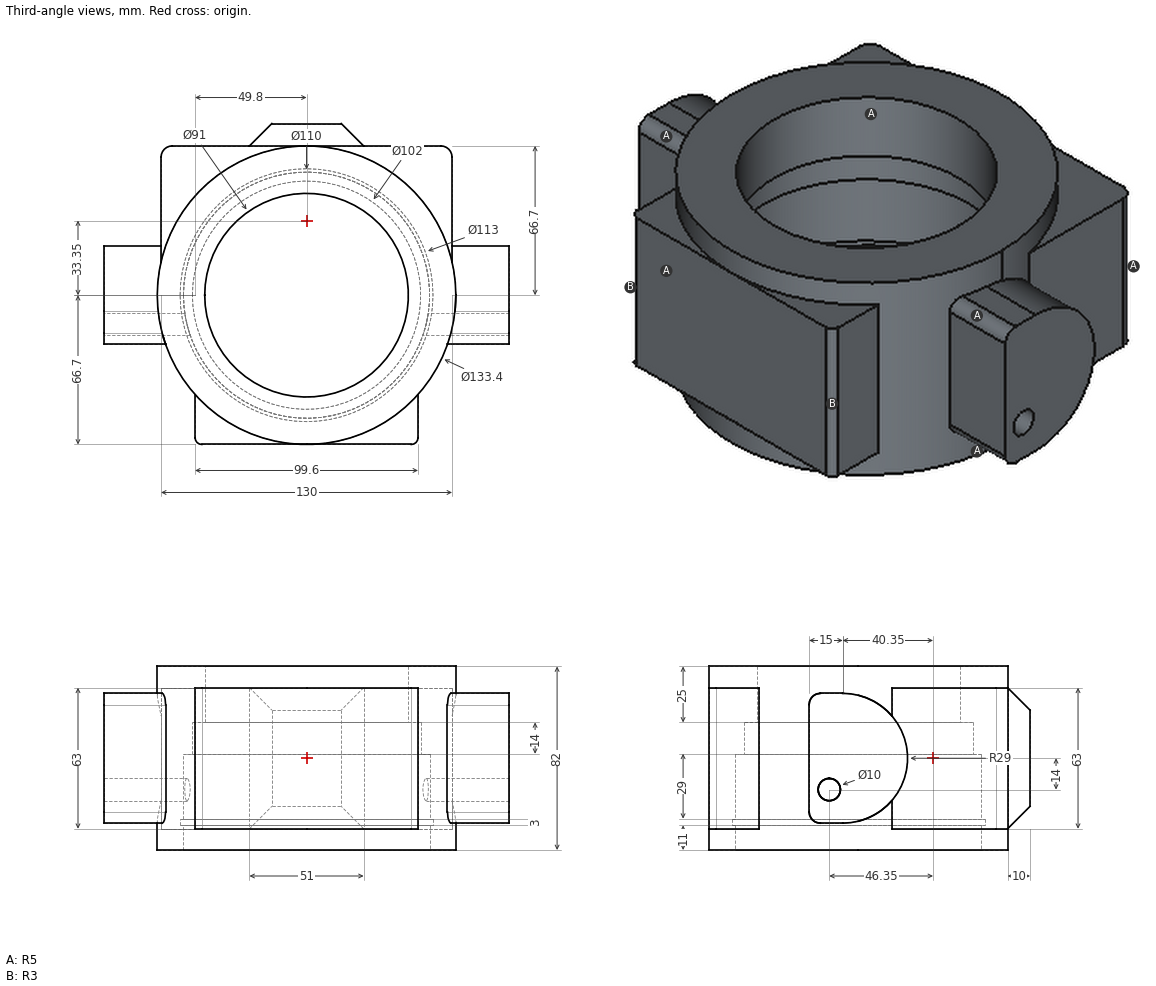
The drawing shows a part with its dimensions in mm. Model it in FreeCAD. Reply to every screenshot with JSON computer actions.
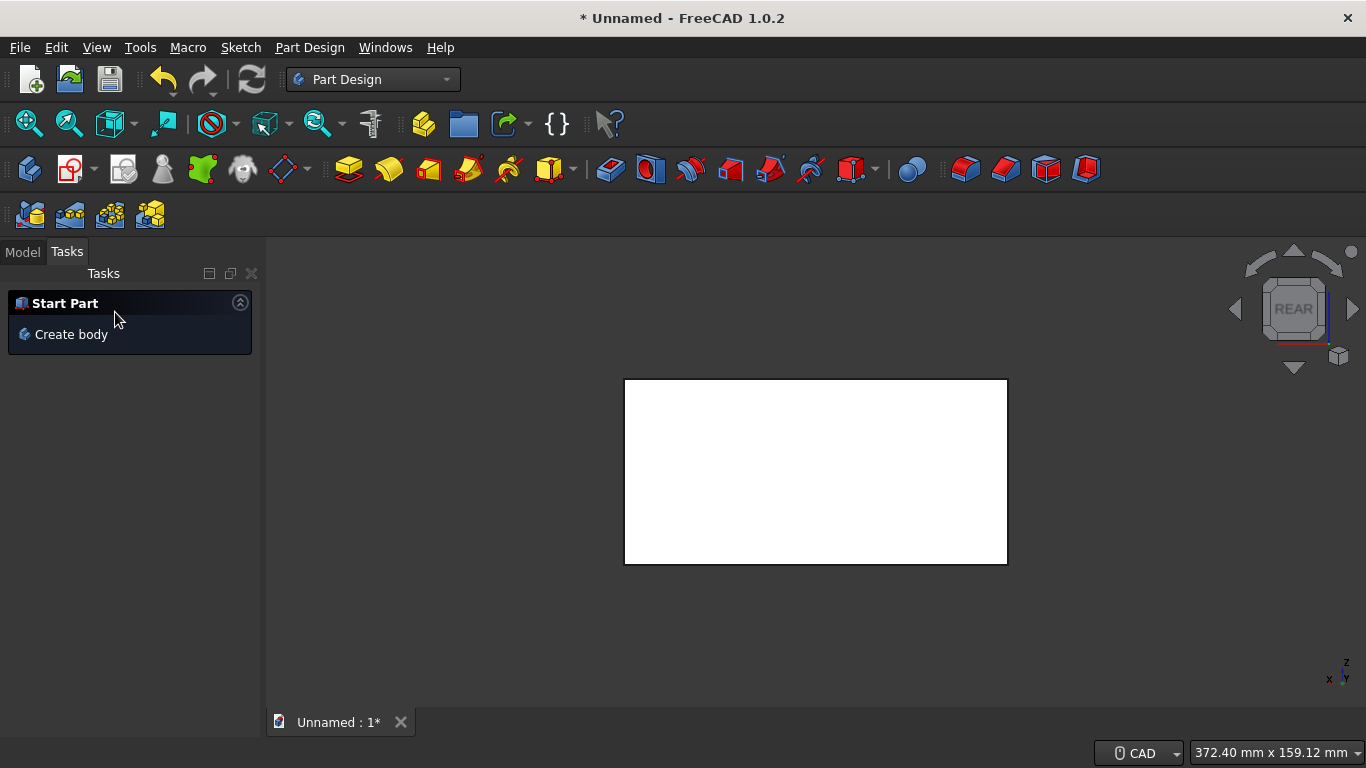
{"action": "key", "text": "v f"}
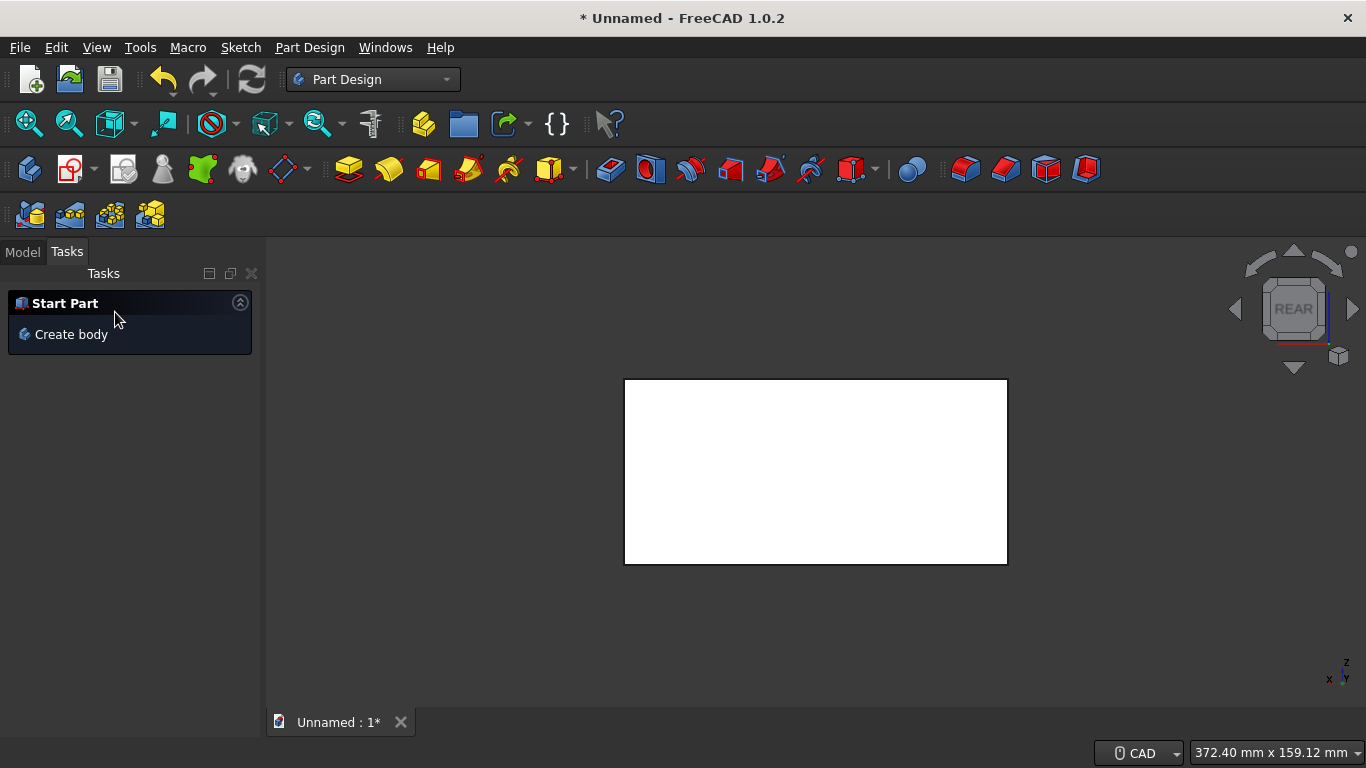
{"action": "left_click", "coordinate": [761, 471]}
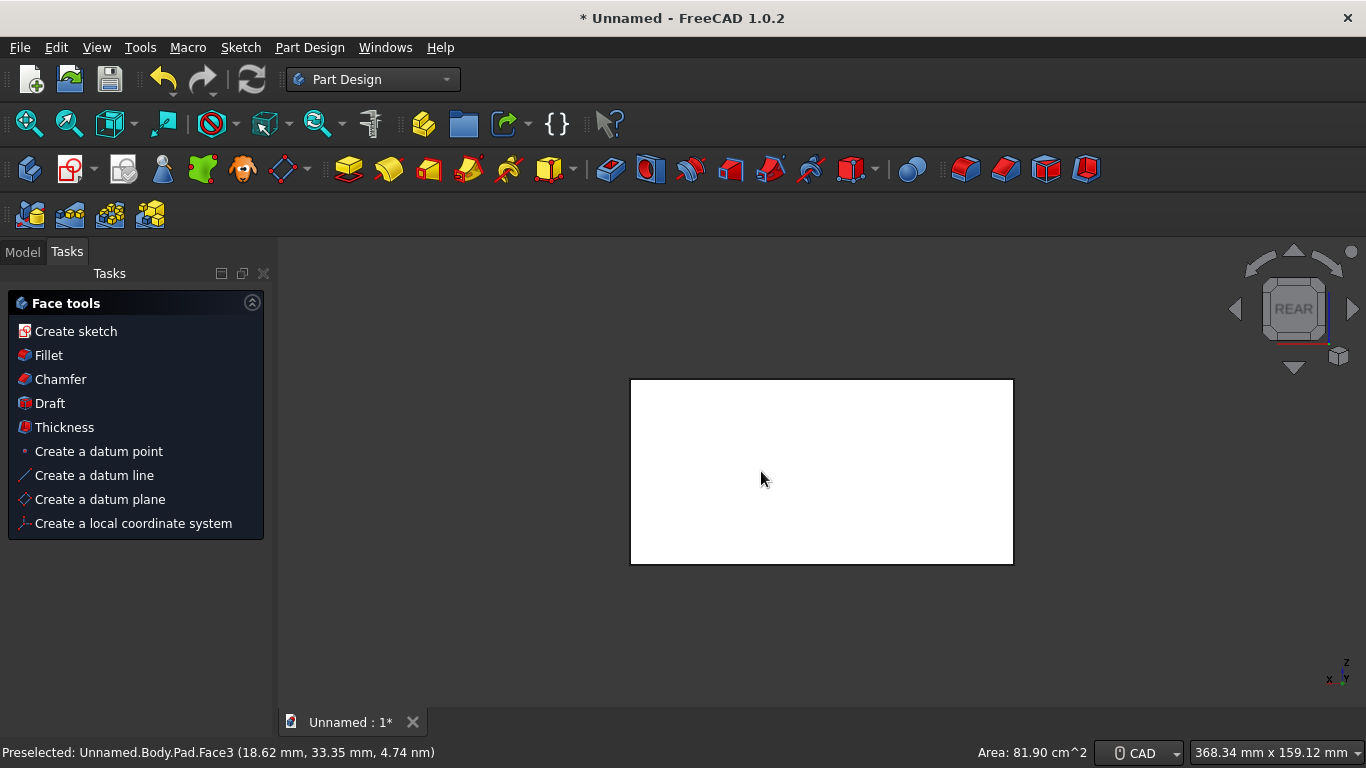
{"action": "left_click", "coordinate": [70, 170]}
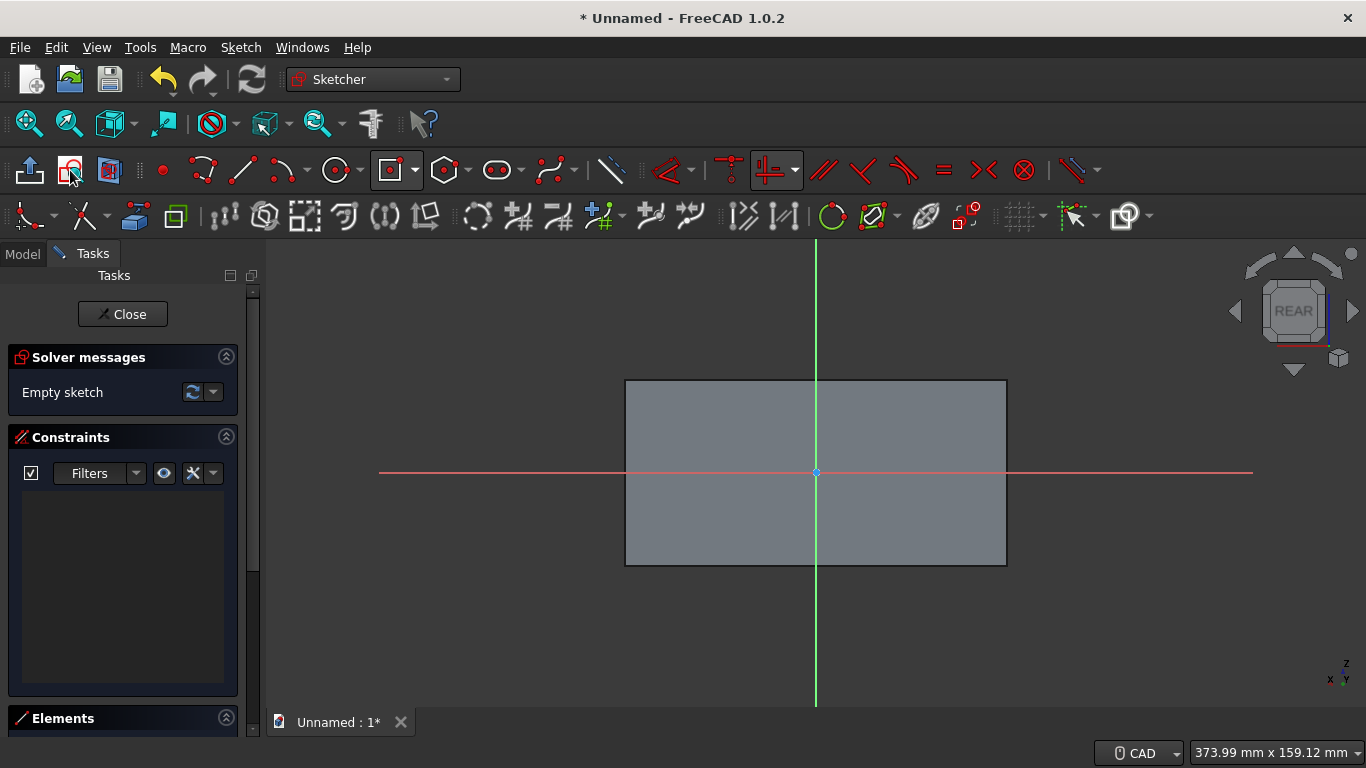
{"action": "scroll", "coordinate": [955, 473], "scroll_direction": "up", "scroll_amount": 2}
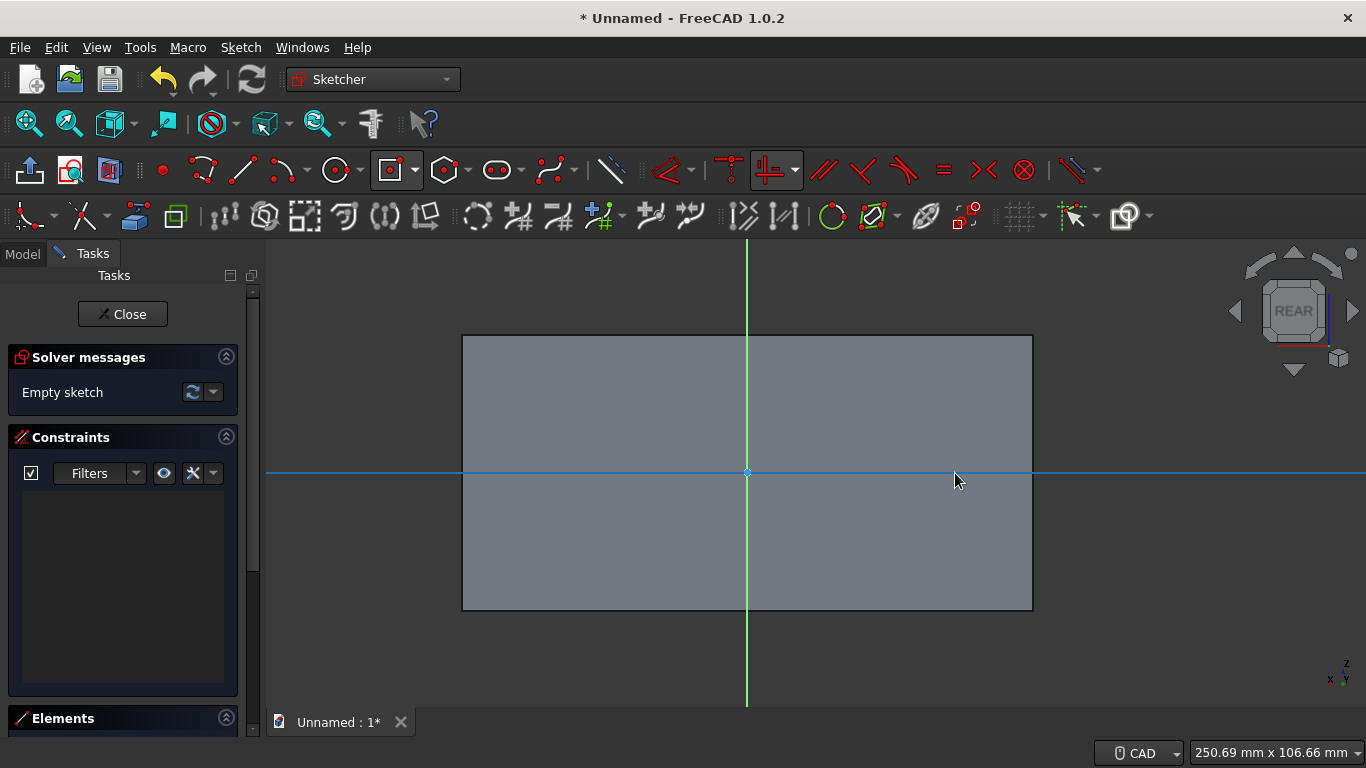
{"action": "key", "text": "g v"}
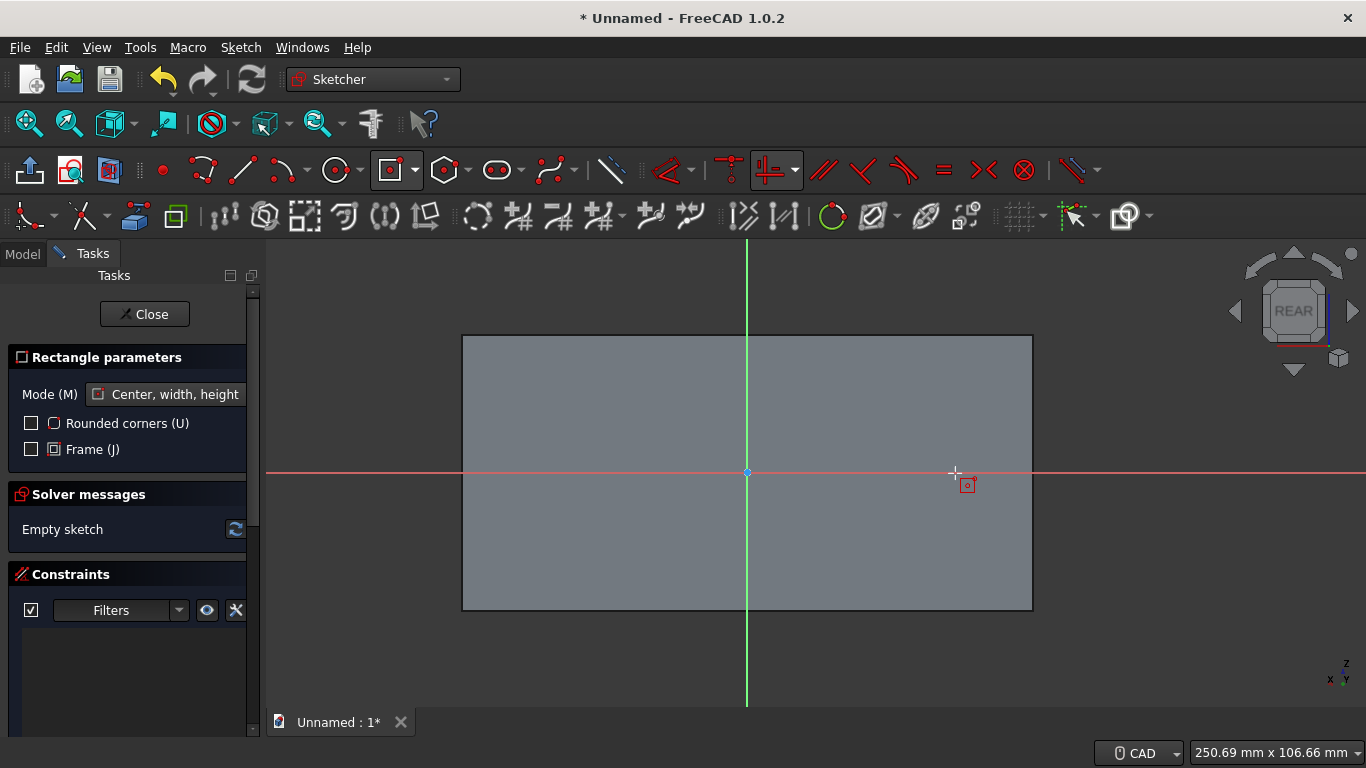
{"action": "left_click", "coordinate": [747, 473]}
{"action": "left_click", "coordinate": [859, 335]}
{"action": "key", "text": "Escape"}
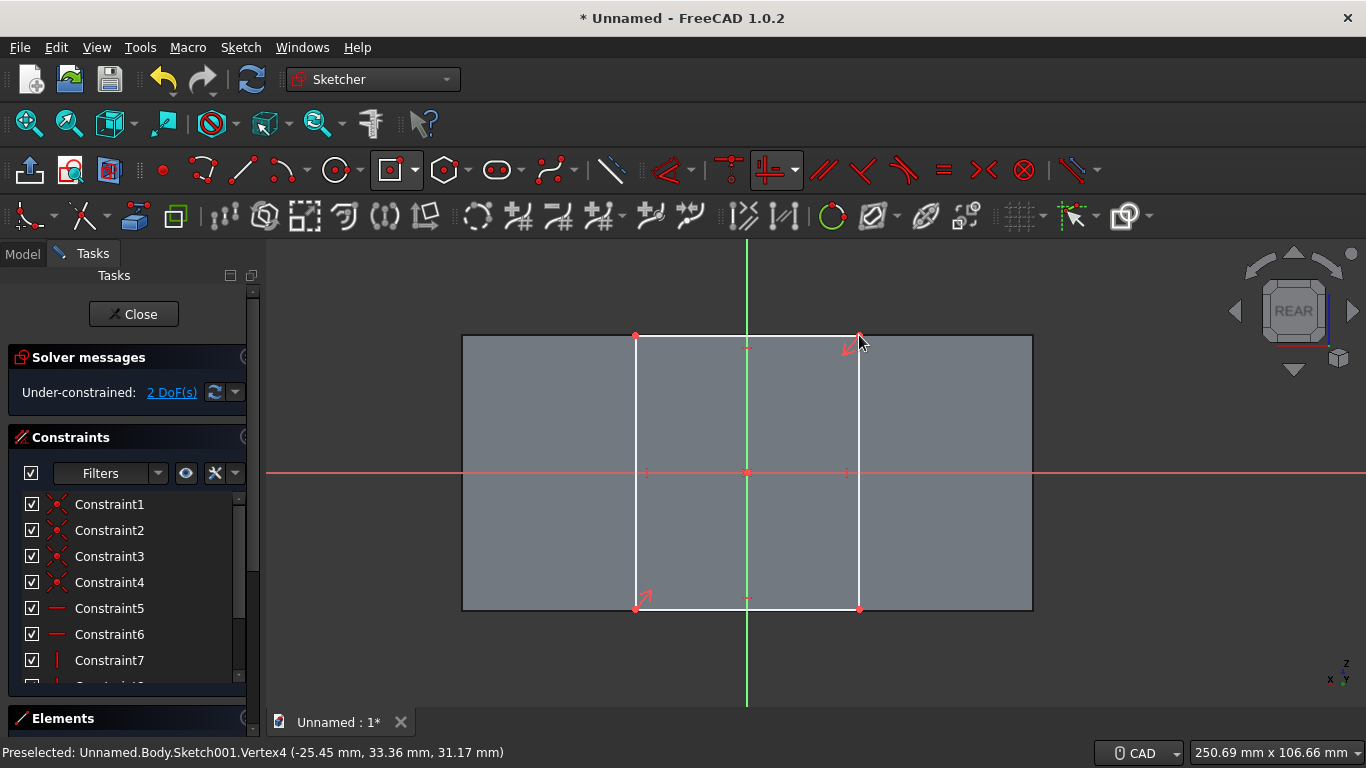
{"action": "left_click", "coordinate": [666, 170]}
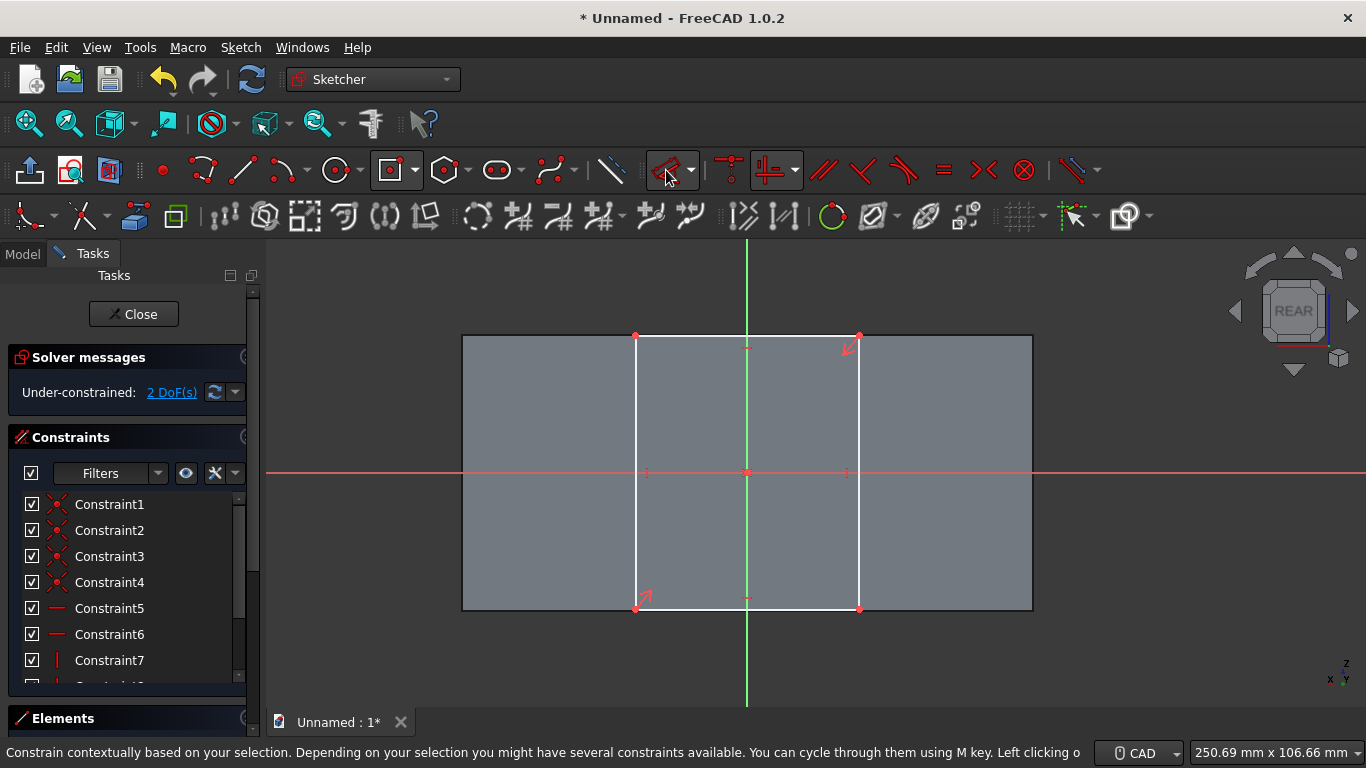
{"action": "left_click", "coordinate": [703, 610]}
{"action": "left_click", "coordinate": [696, 644]}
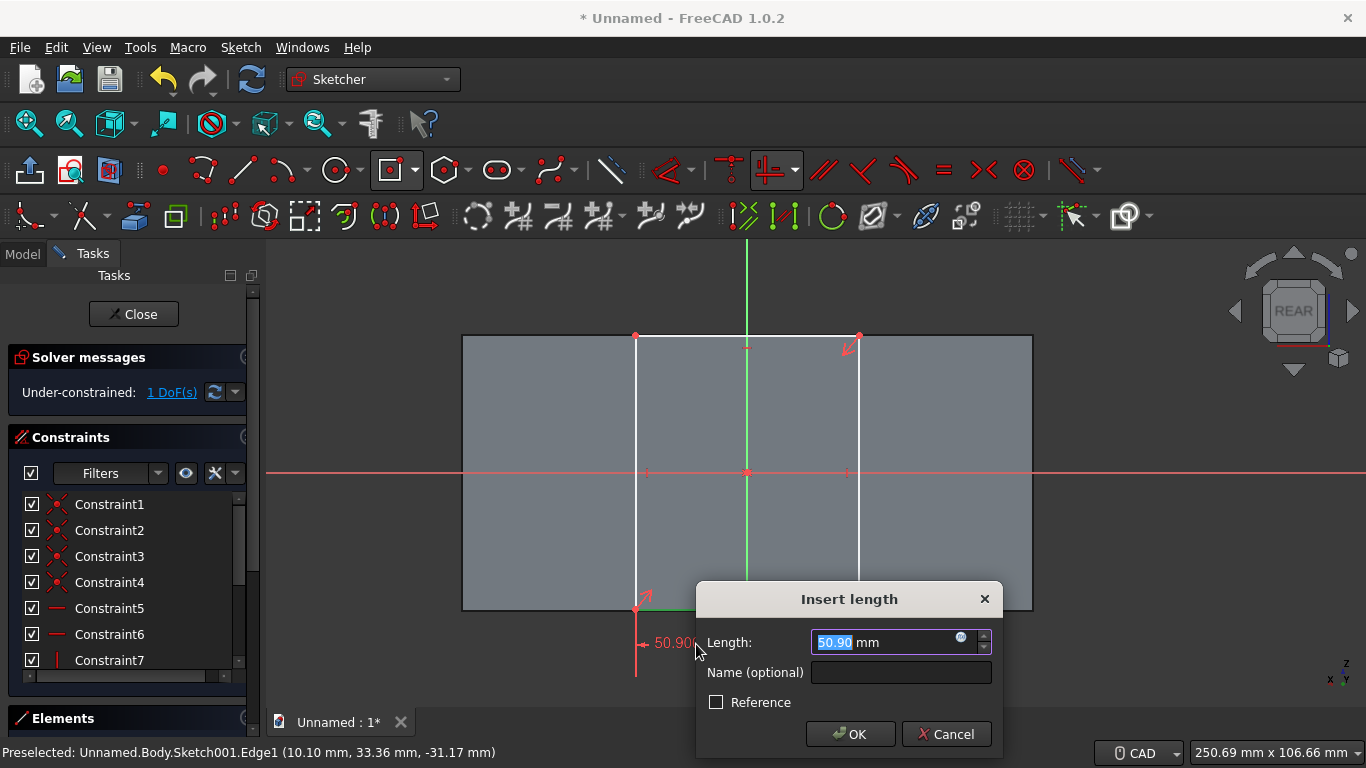
{"action": "type", "text": "51"}
{"action": "key", "text": "Return"}